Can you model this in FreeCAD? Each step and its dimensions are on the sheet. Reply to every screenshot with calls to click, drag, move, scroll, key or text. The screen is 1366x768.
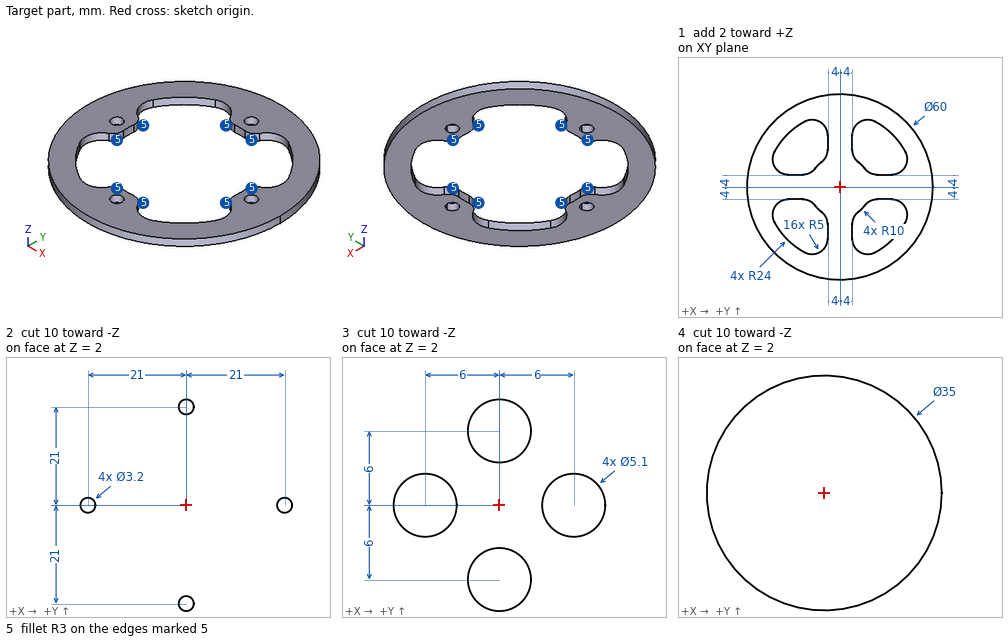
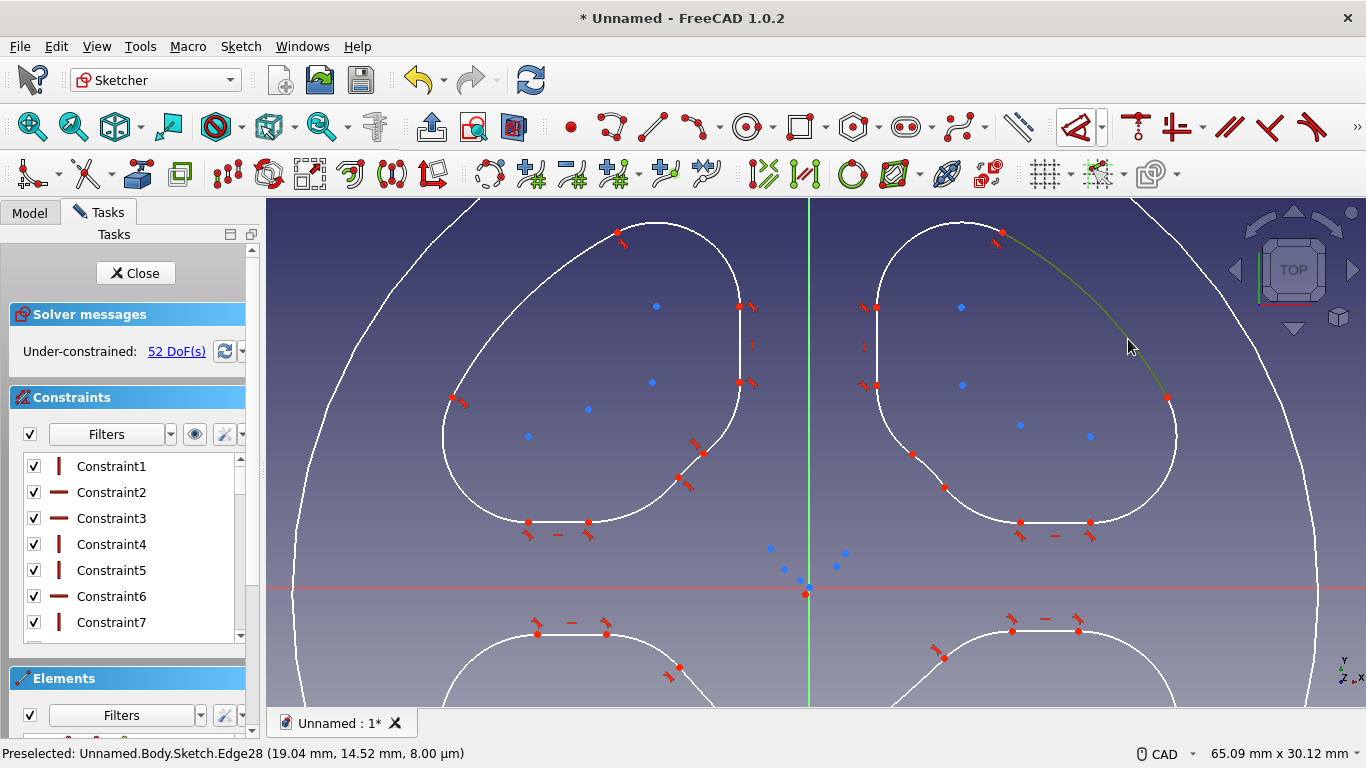
click(1140, 507)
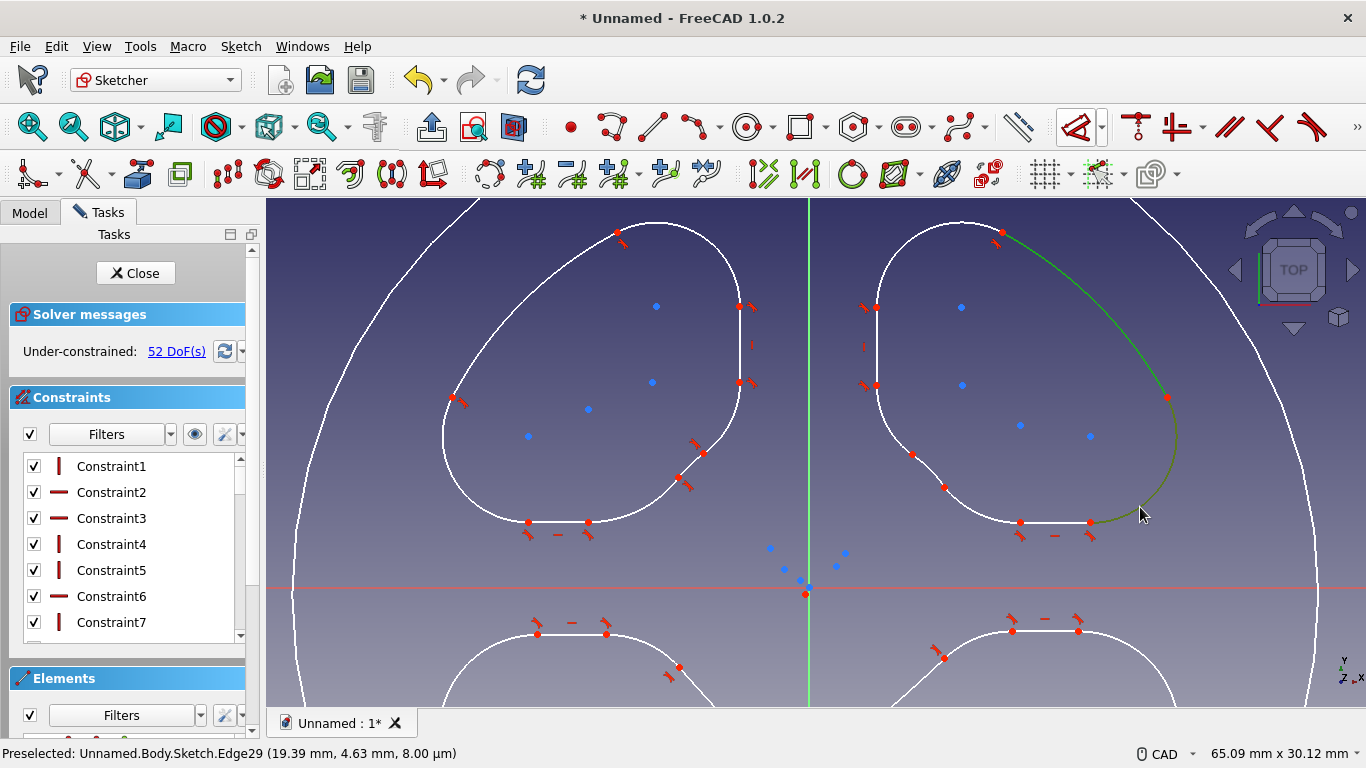
key(t)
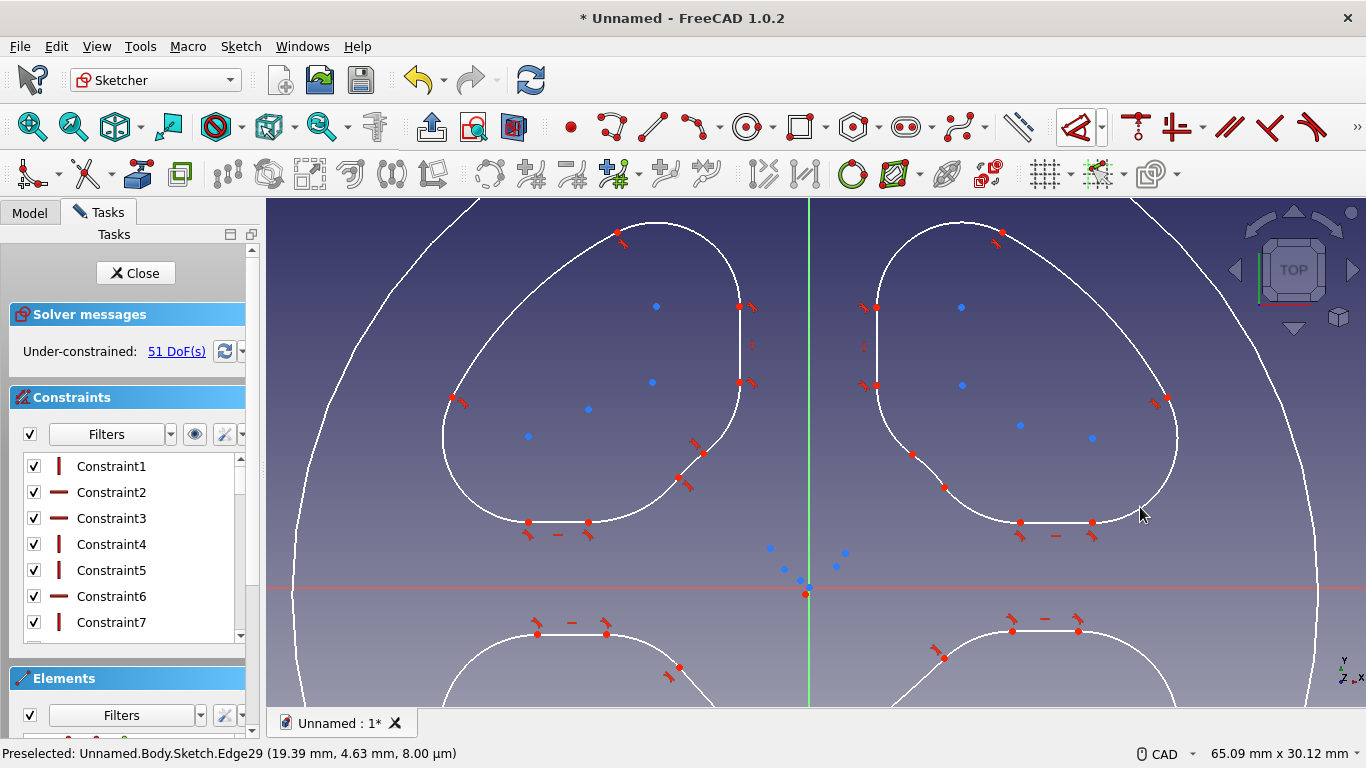
click(964, 505)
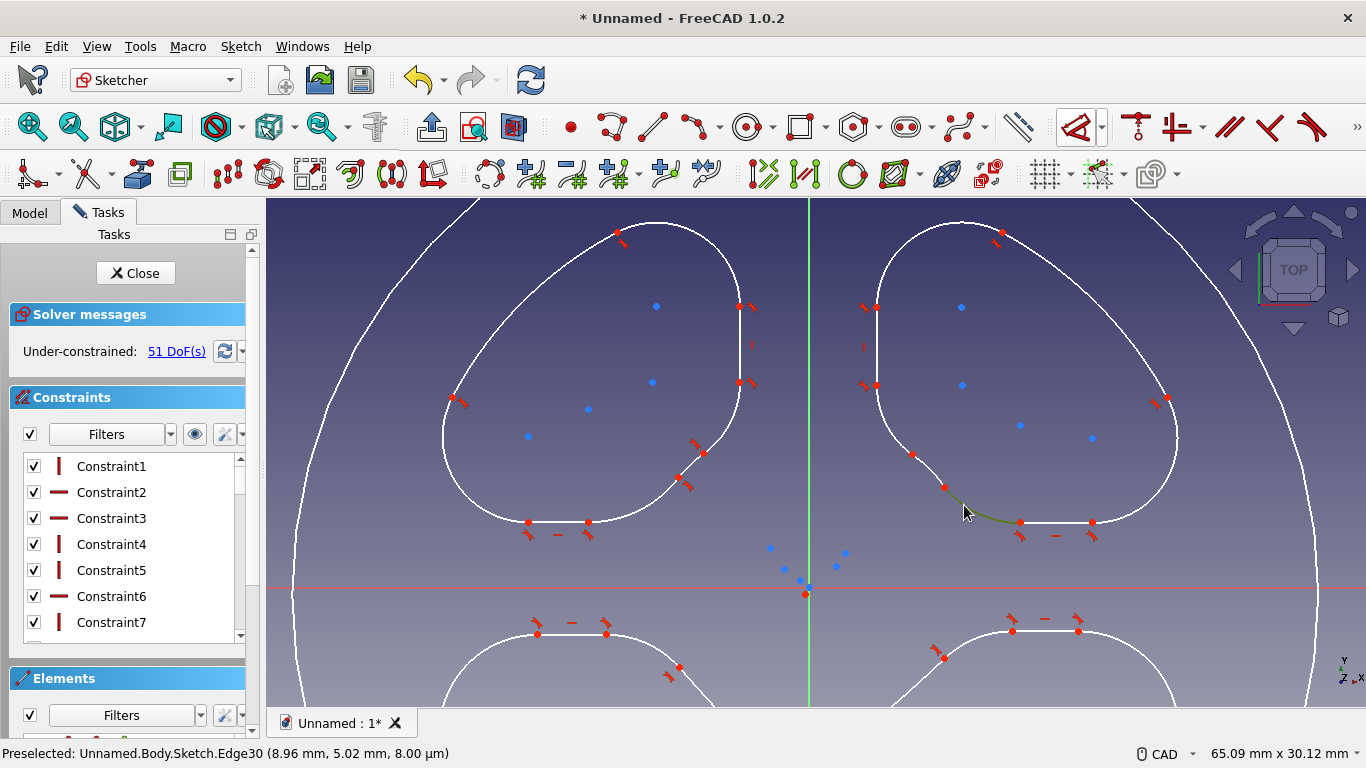
click(936, 476)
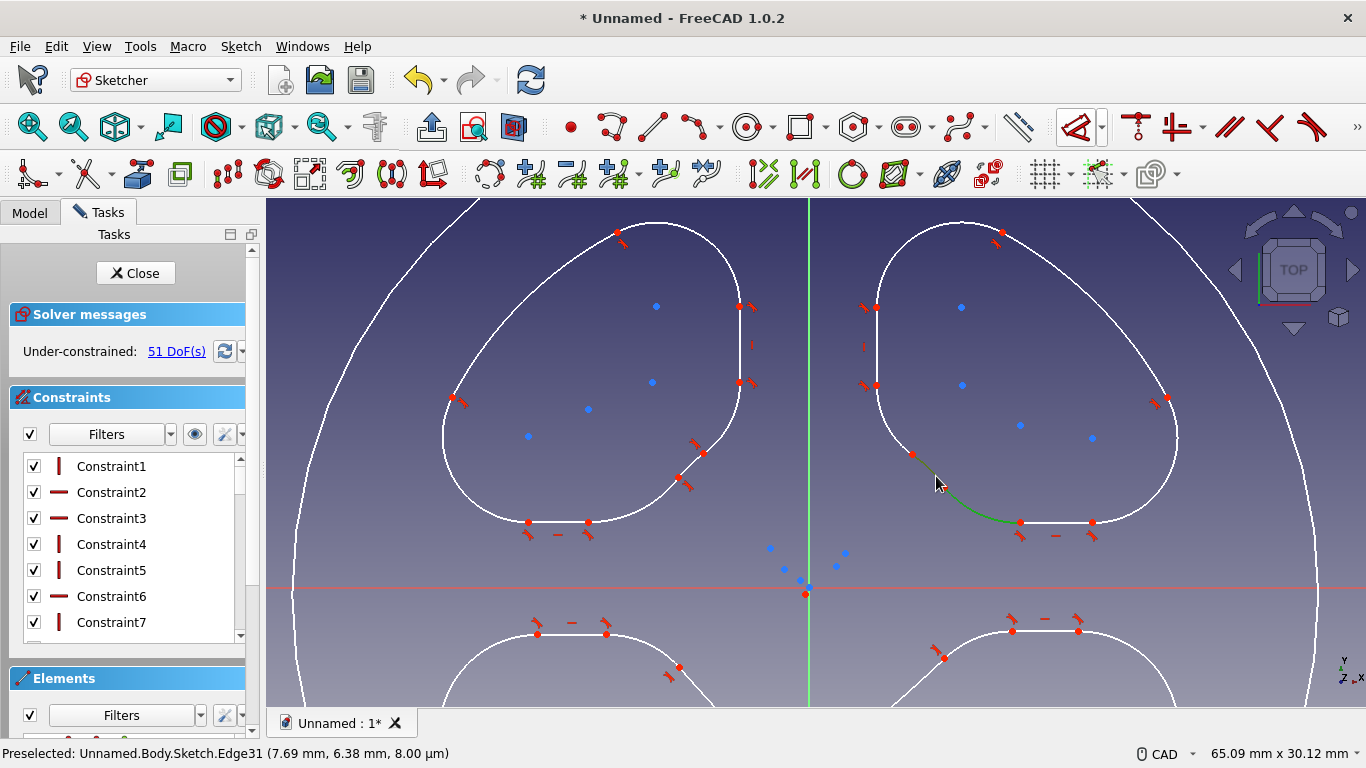
key(t)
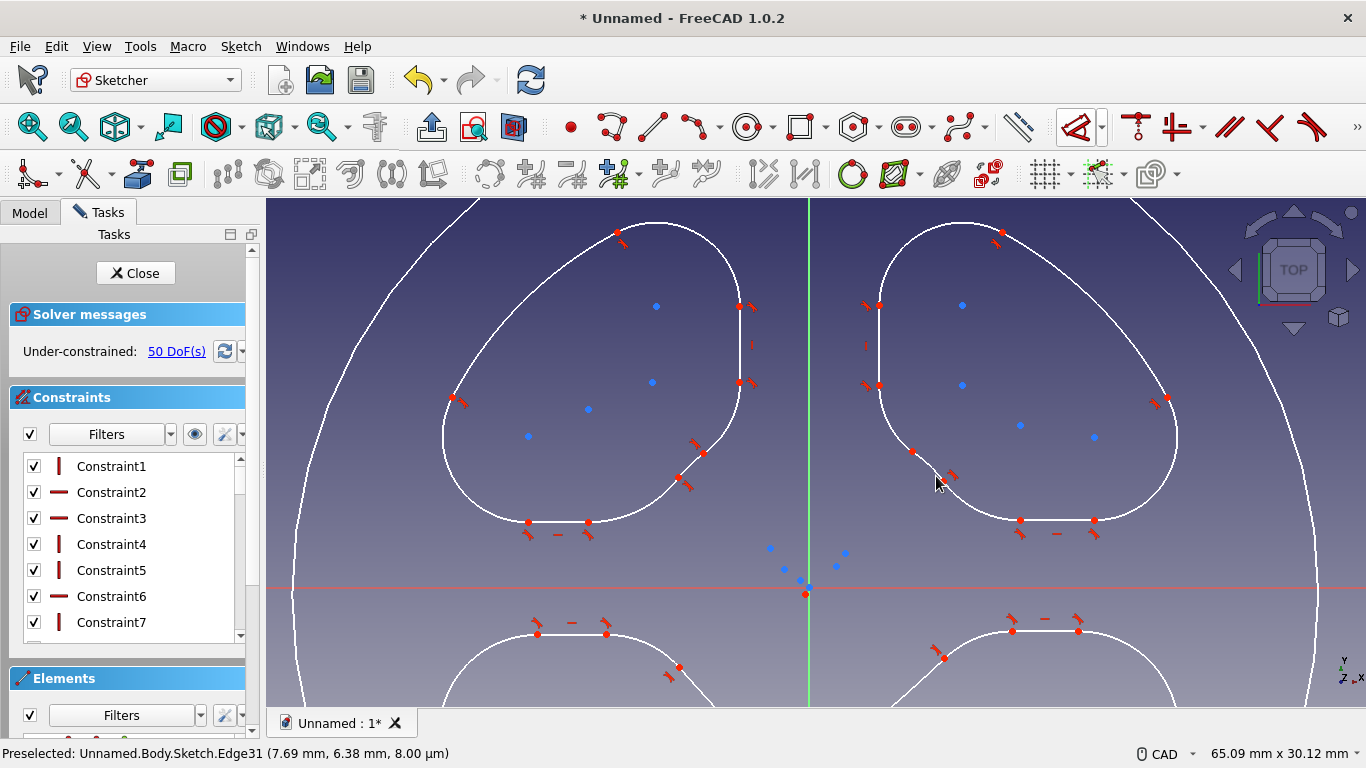
click(935, 471)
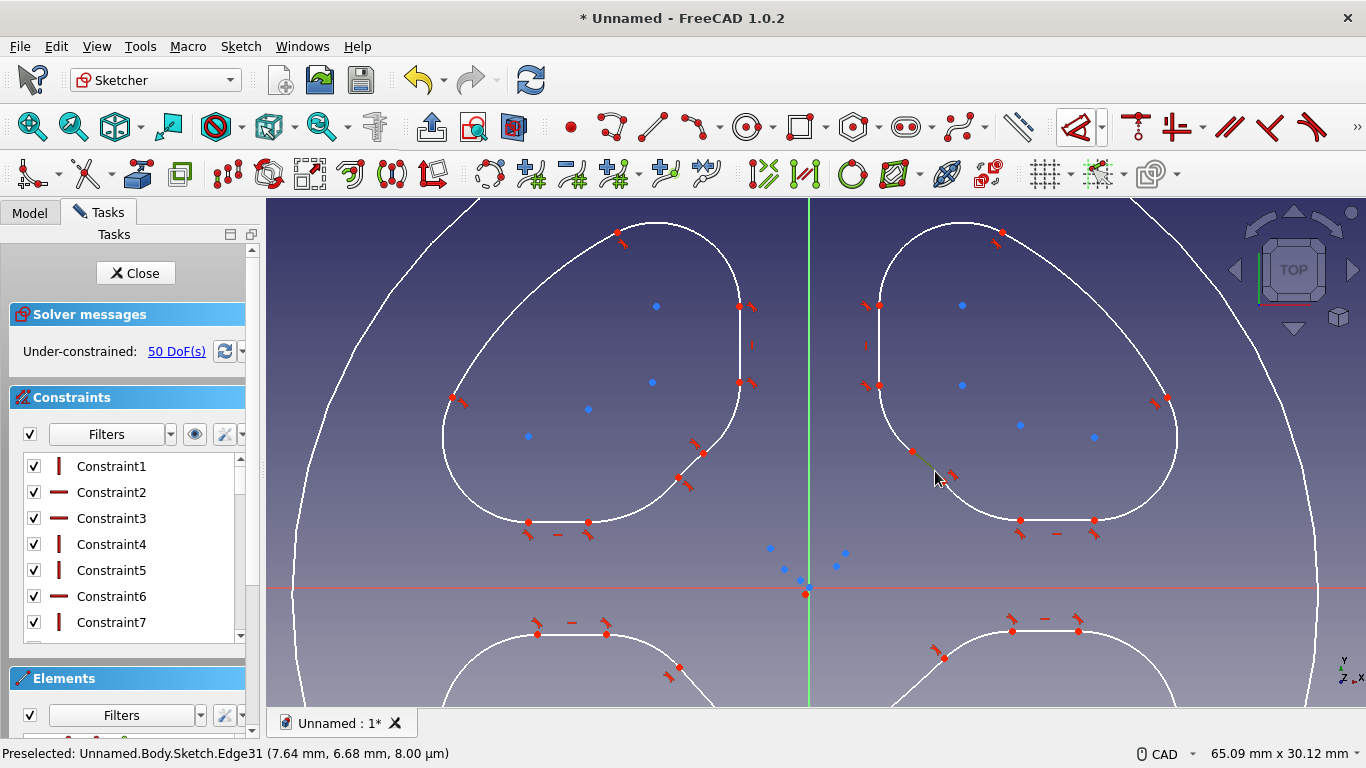
click(883, 408)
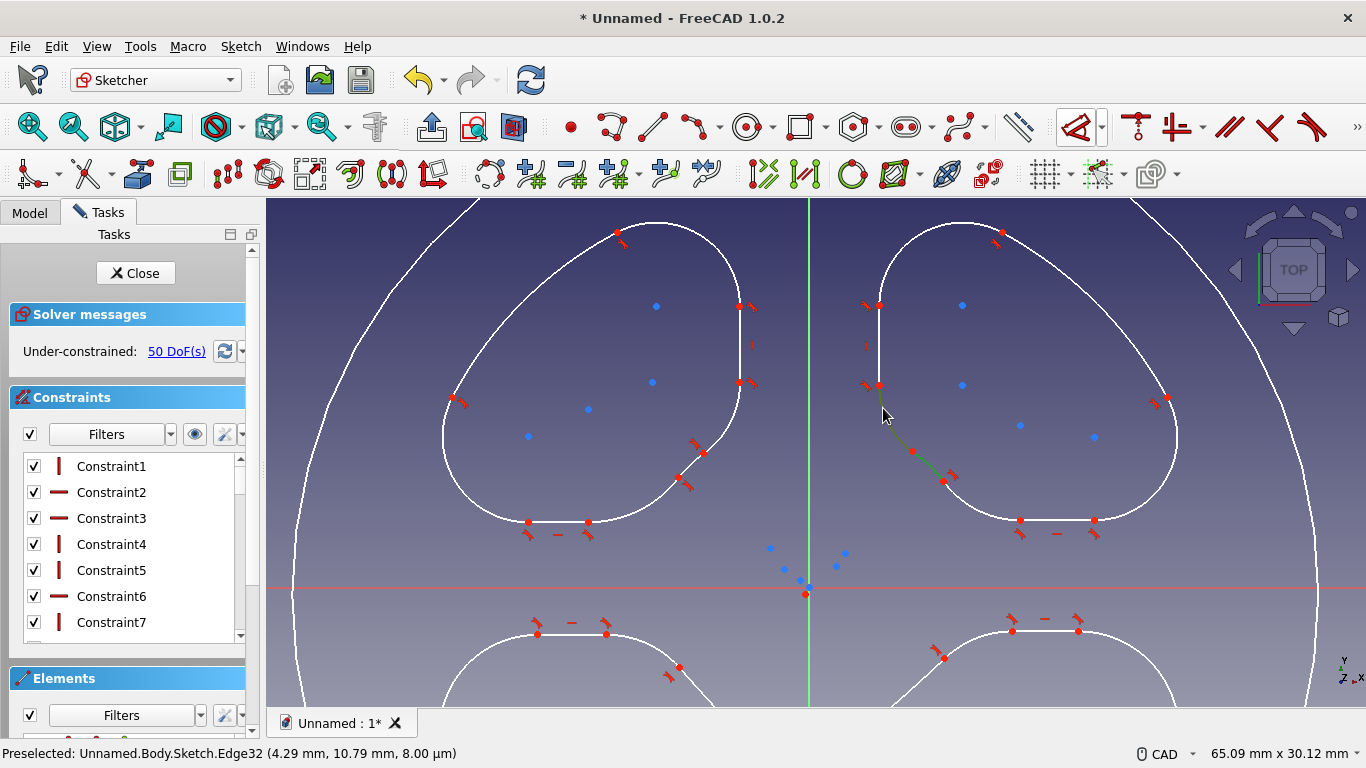
click(1312, 128)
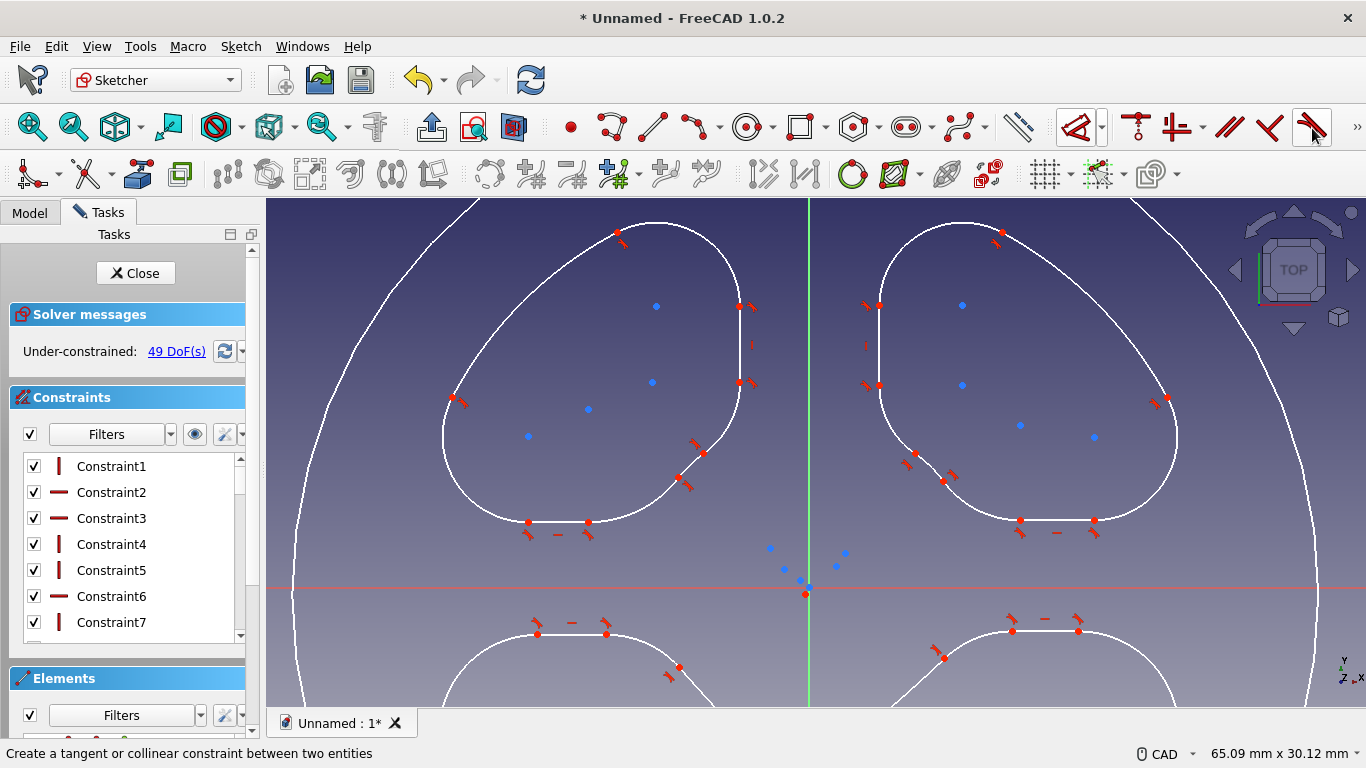
click(1167, 231)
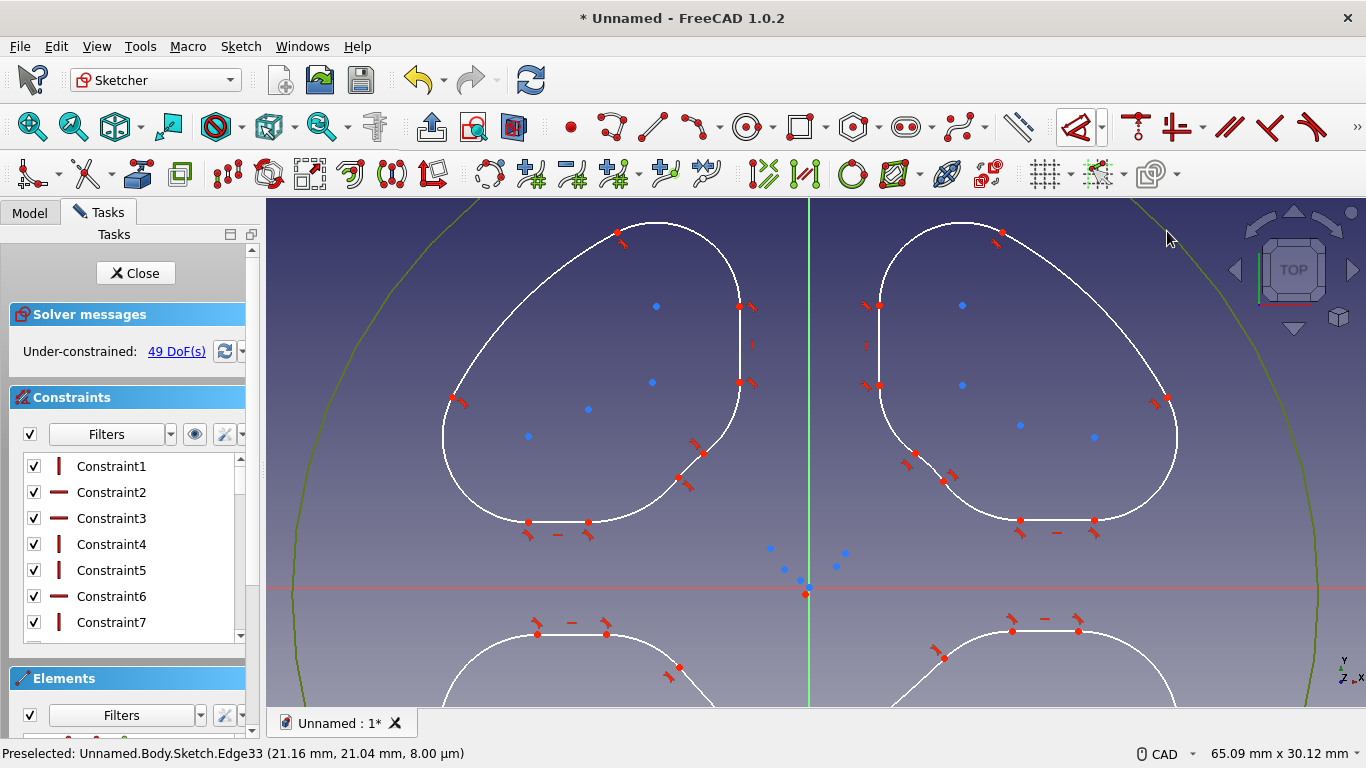
scroll(721, 394, down, 6)